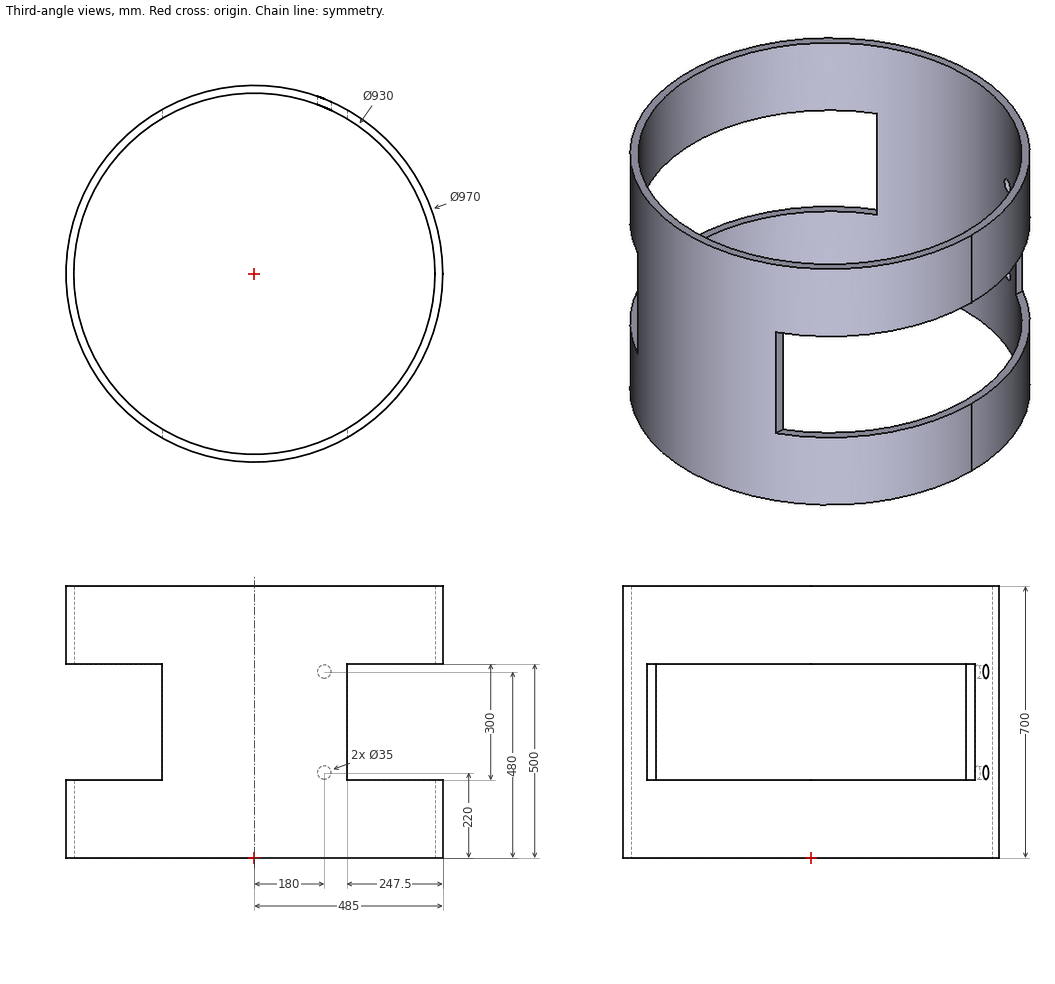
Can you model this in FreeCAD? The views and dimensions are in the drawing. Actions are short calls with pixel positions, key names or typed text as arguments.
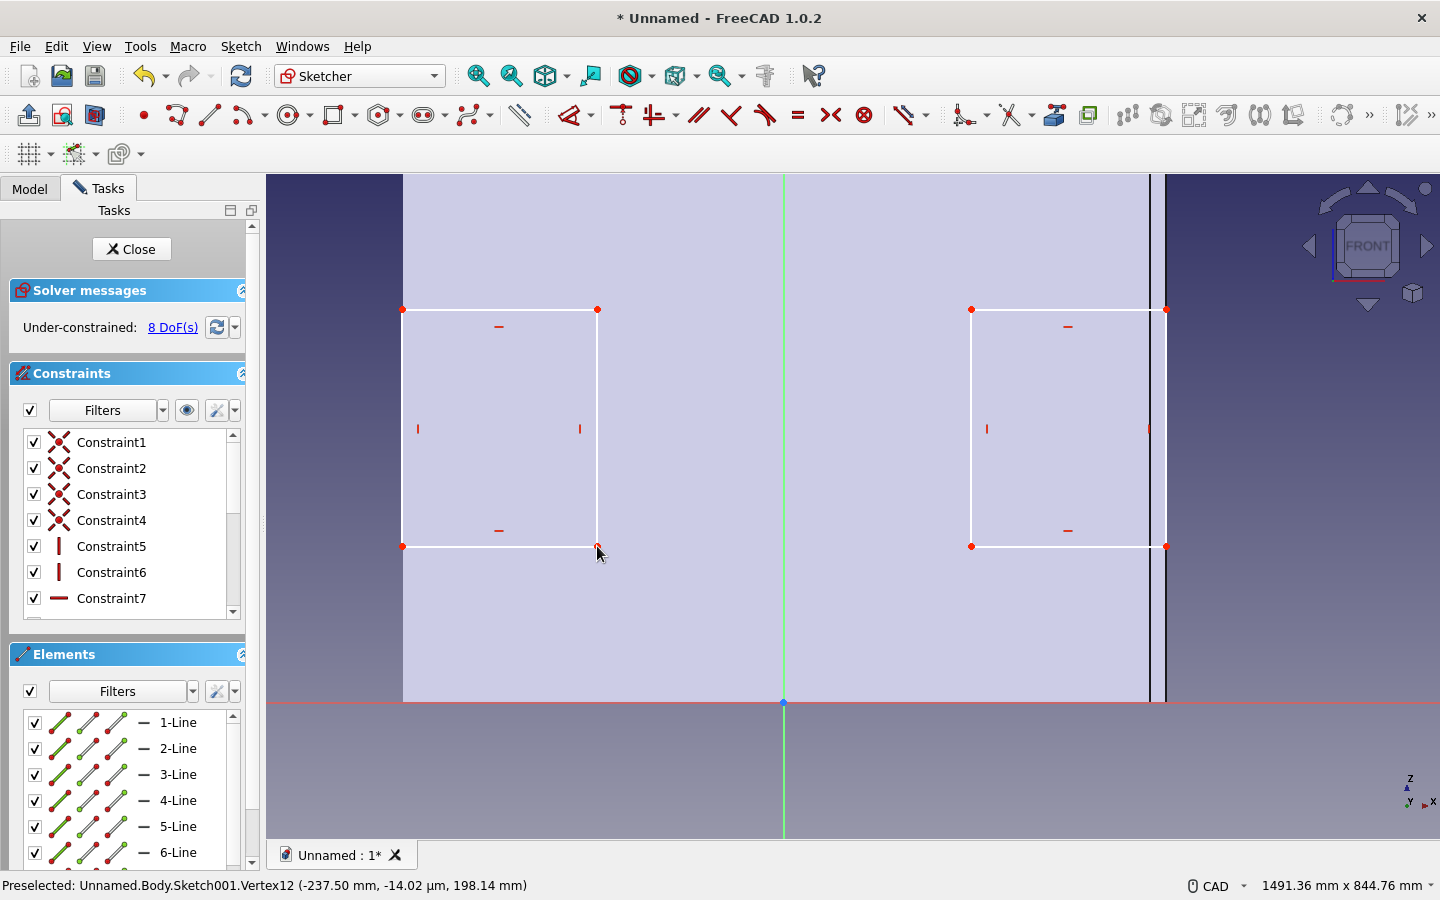
click(1166, 310)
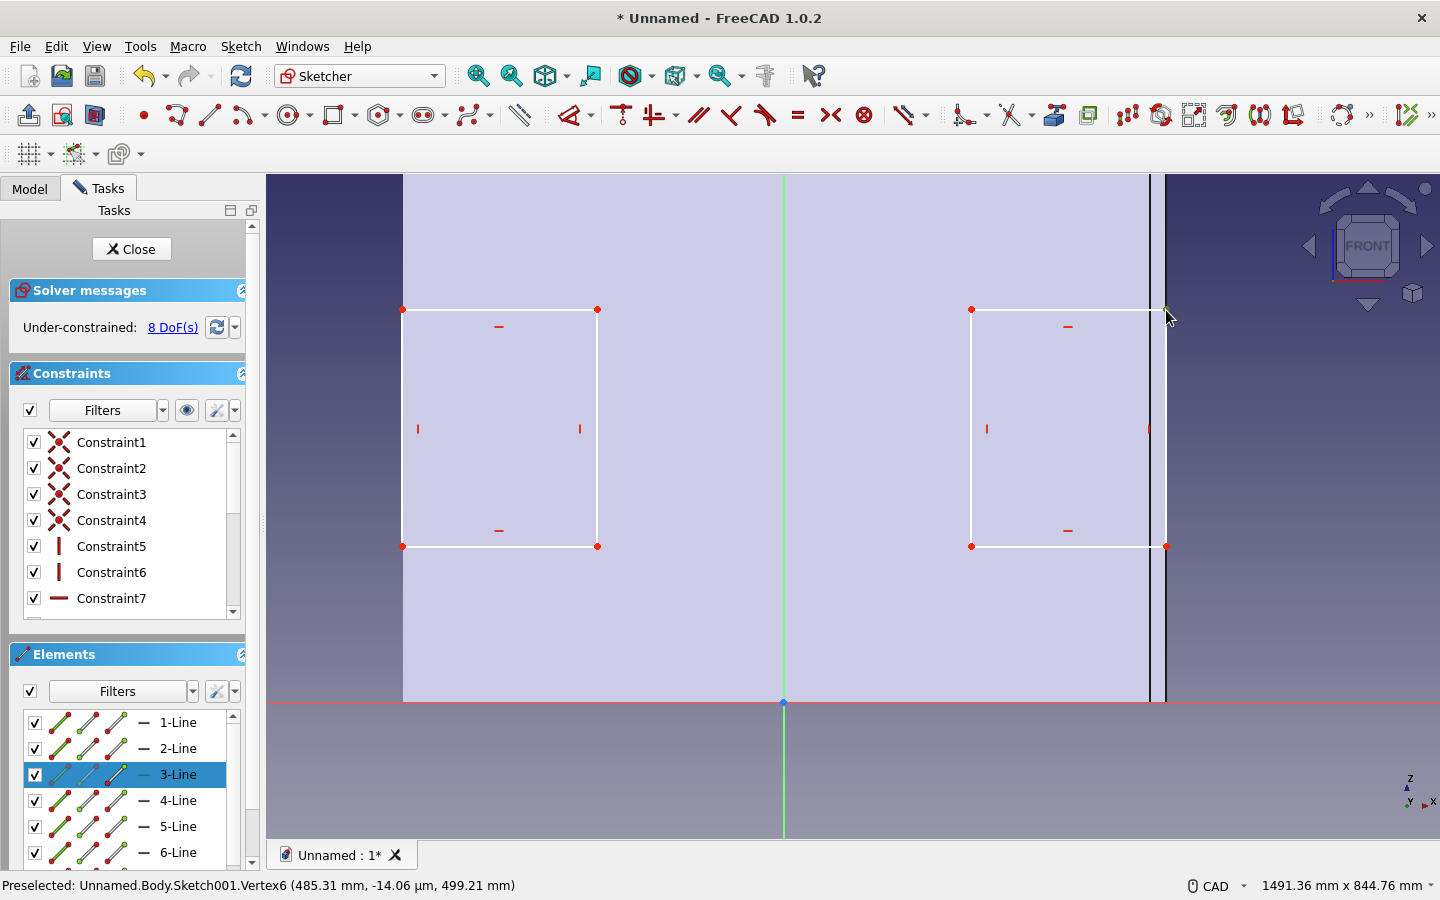
click(402, 310)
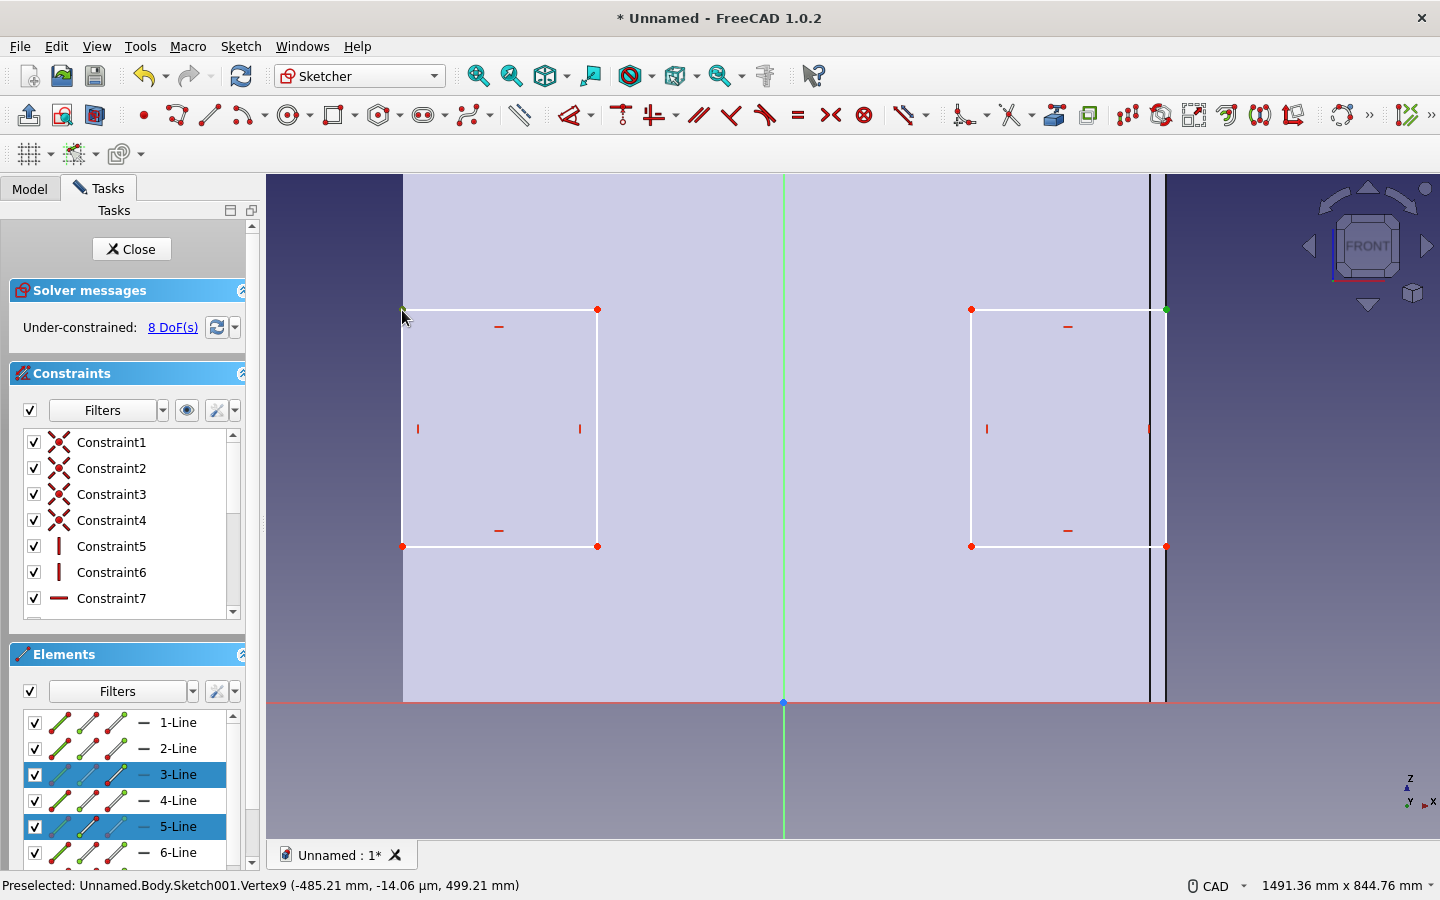
click(784, 768)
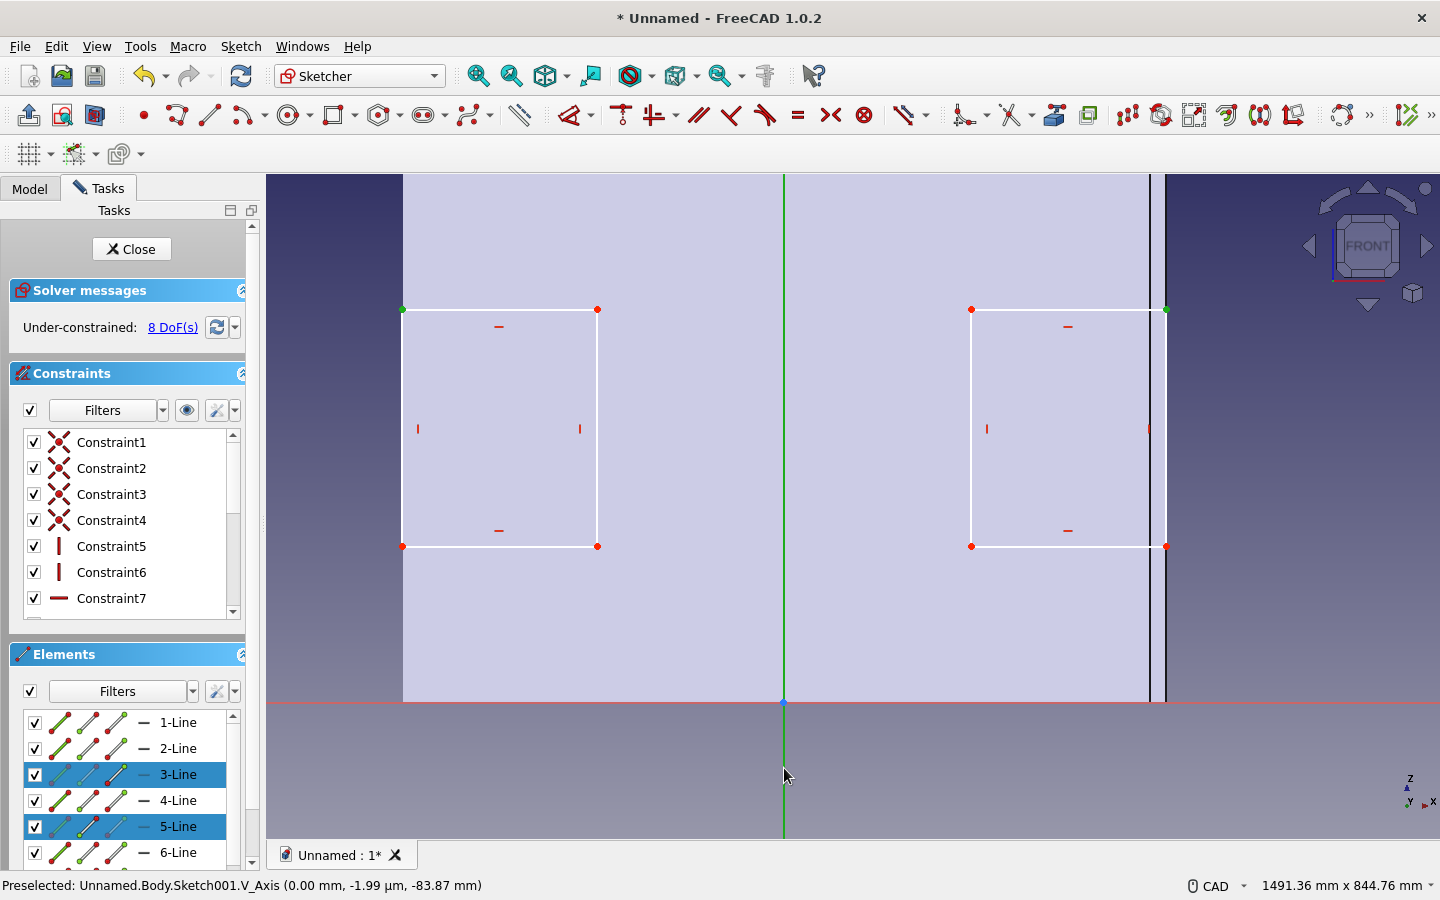
click(831, 116)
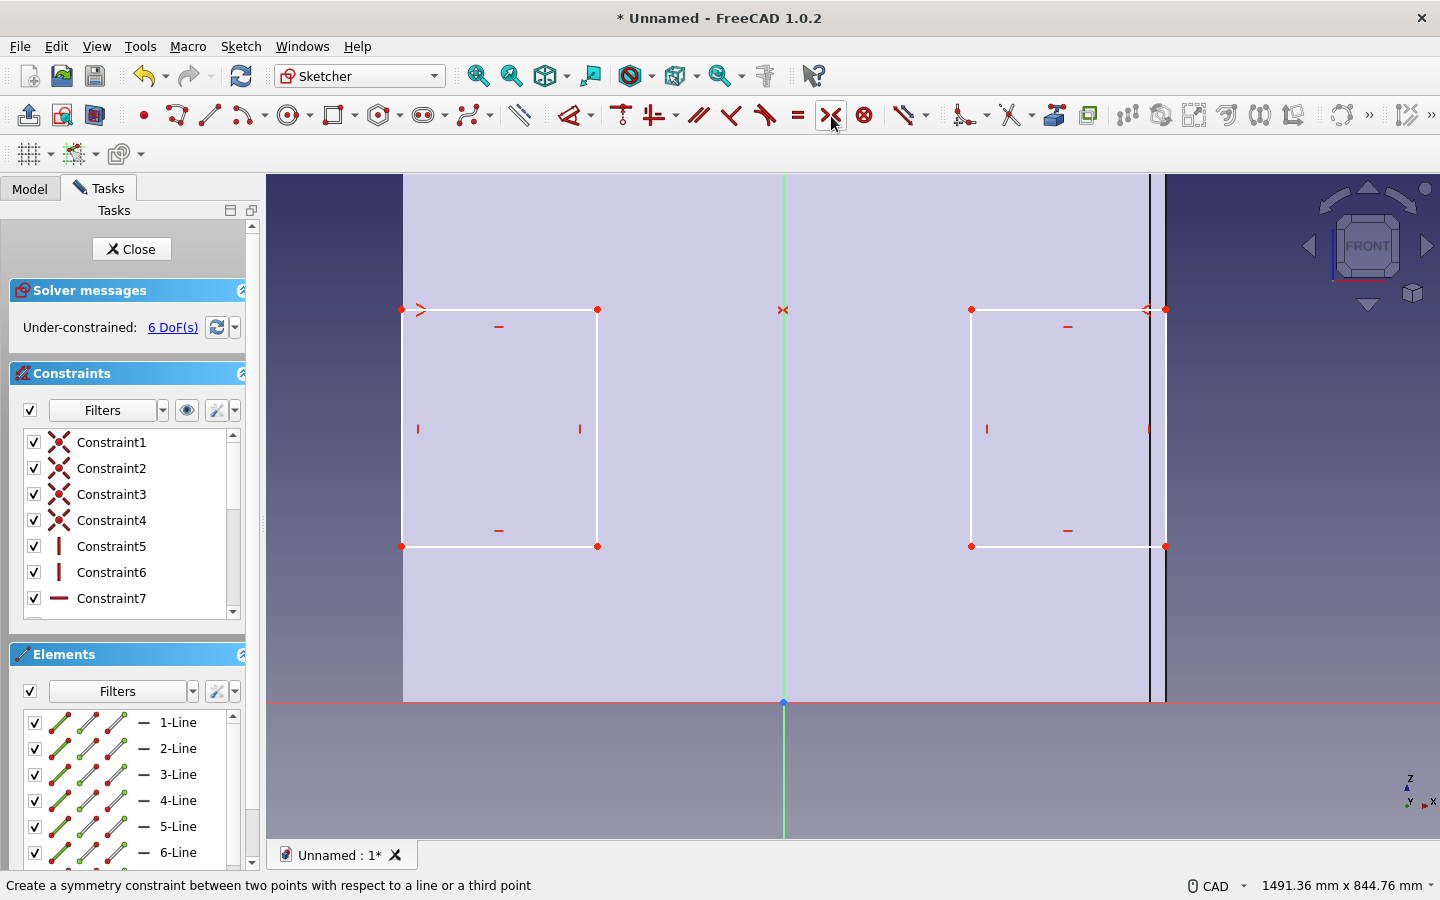
click(971, 547)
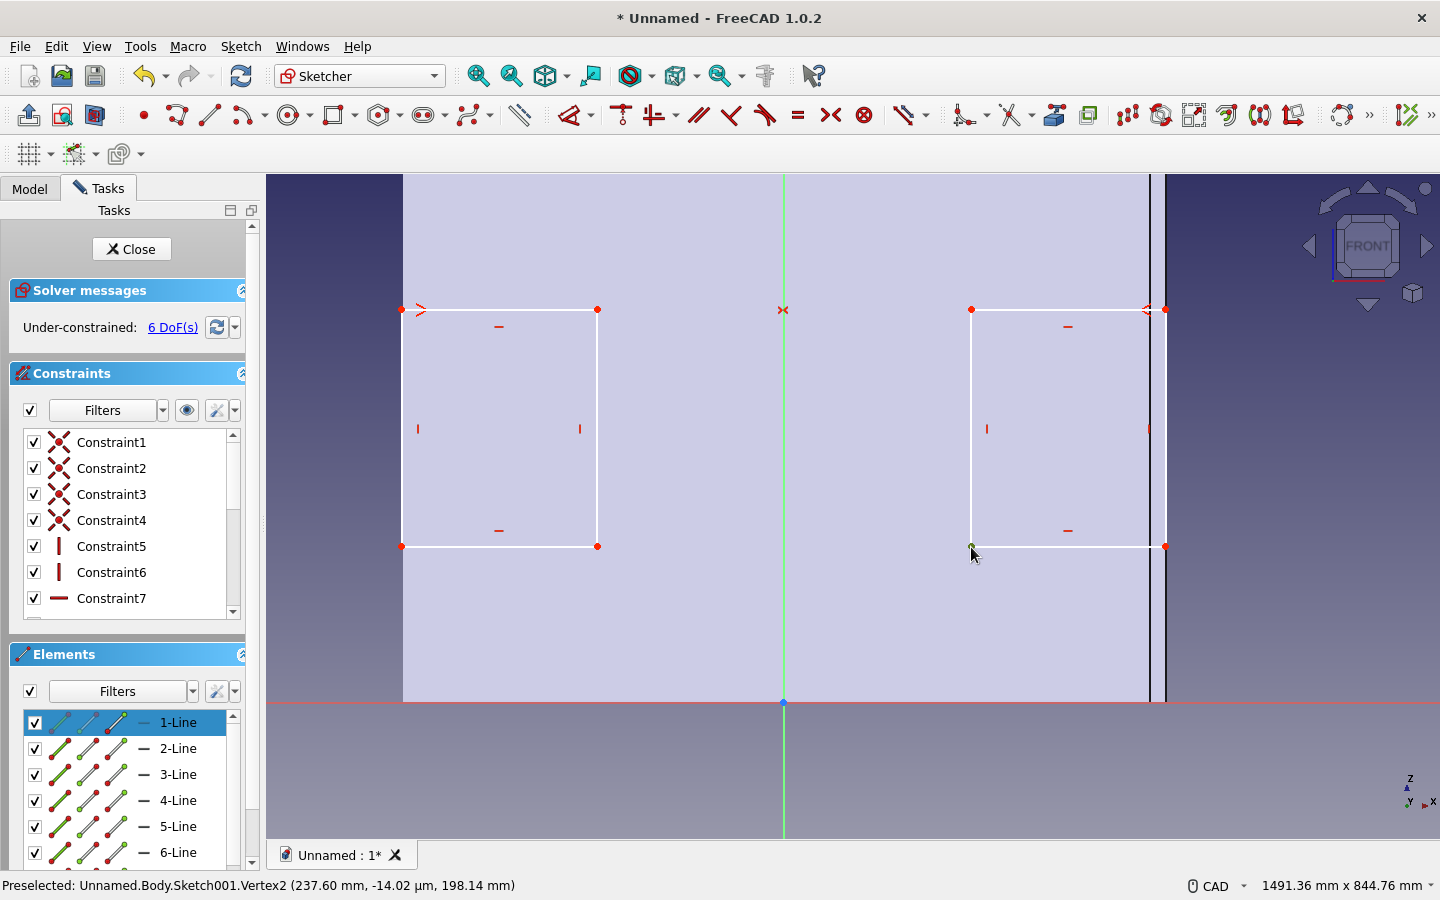
click(597, 547)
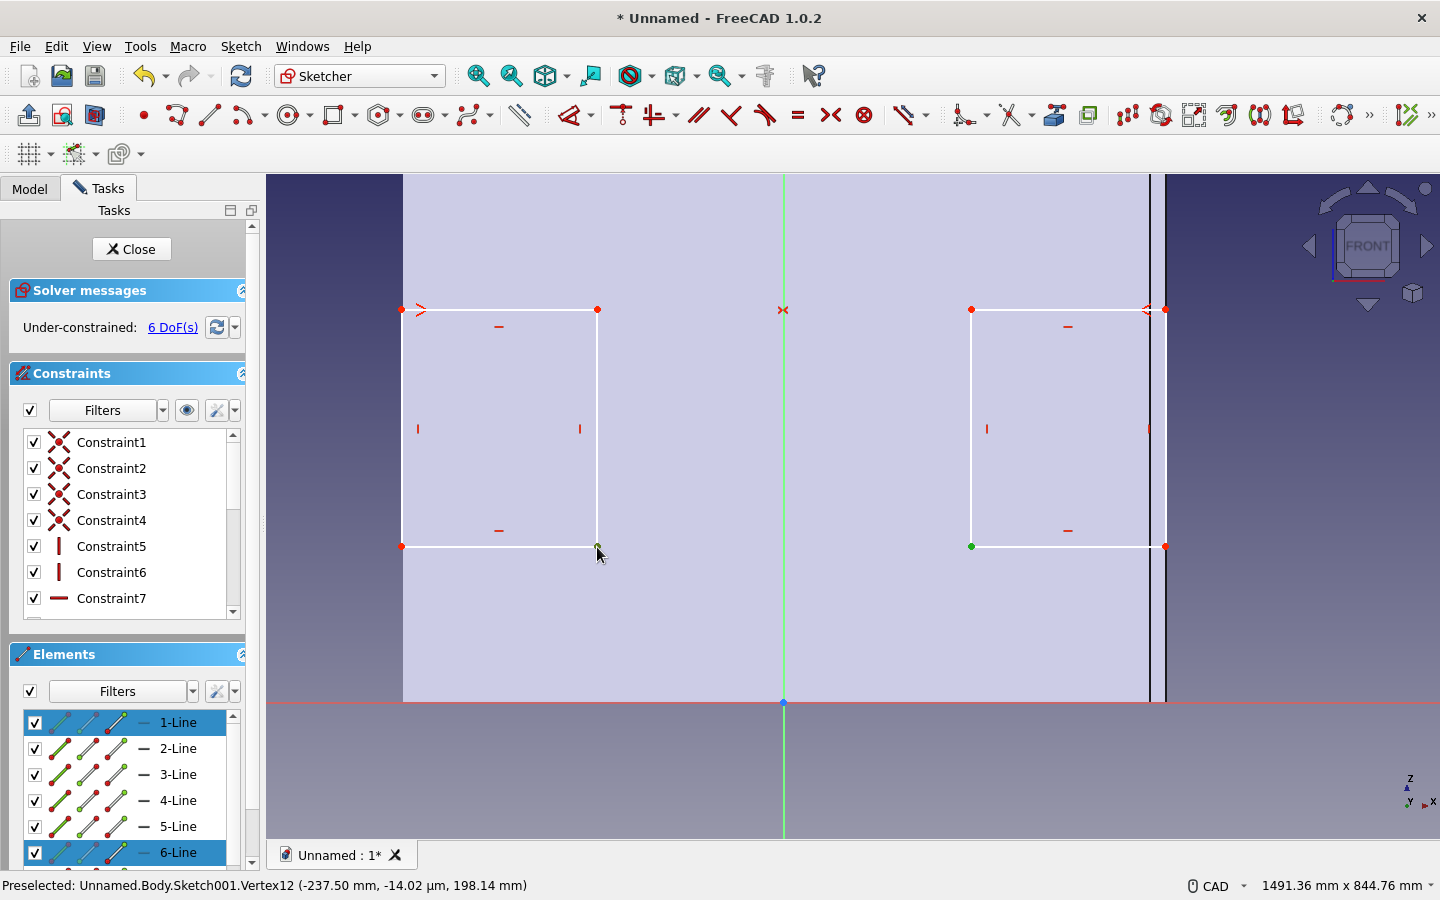
click(784, 768)